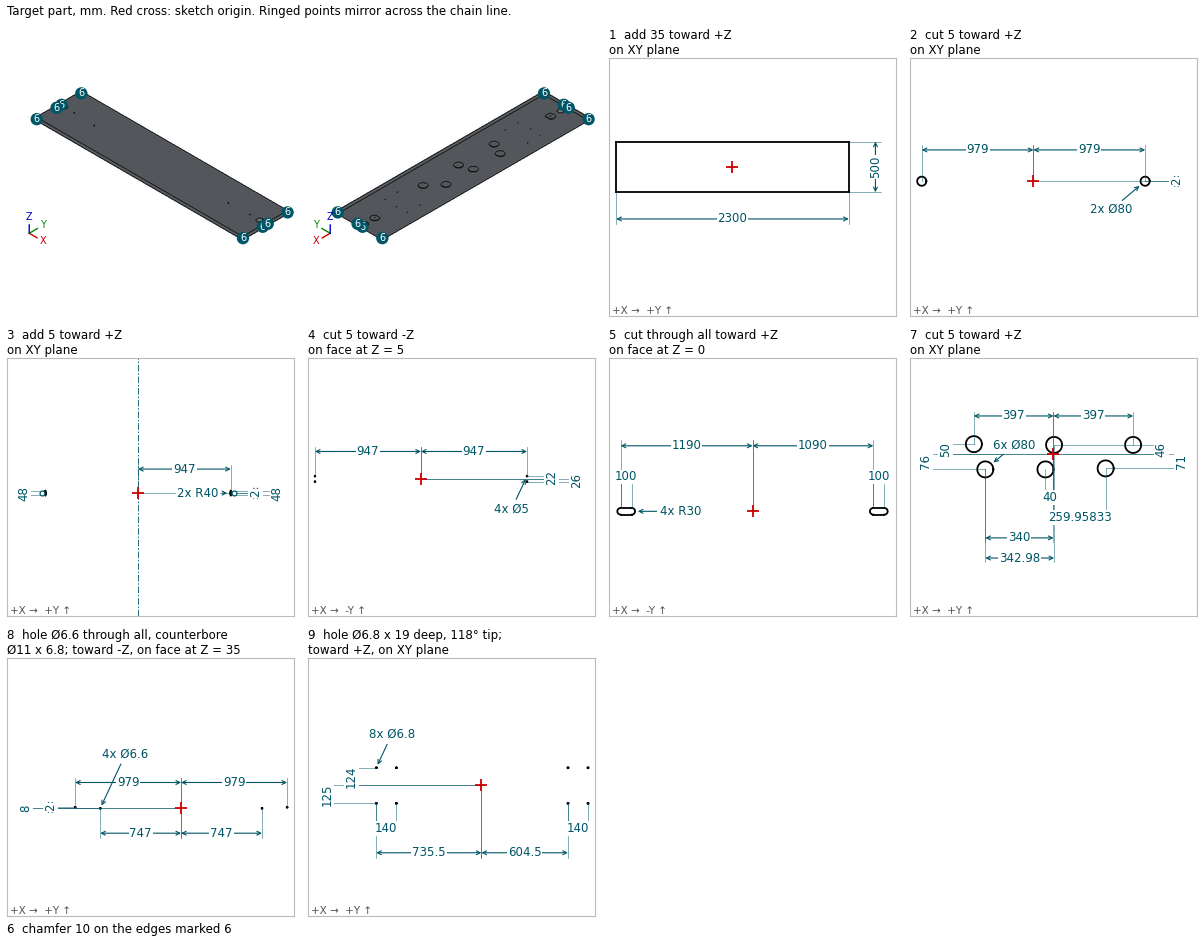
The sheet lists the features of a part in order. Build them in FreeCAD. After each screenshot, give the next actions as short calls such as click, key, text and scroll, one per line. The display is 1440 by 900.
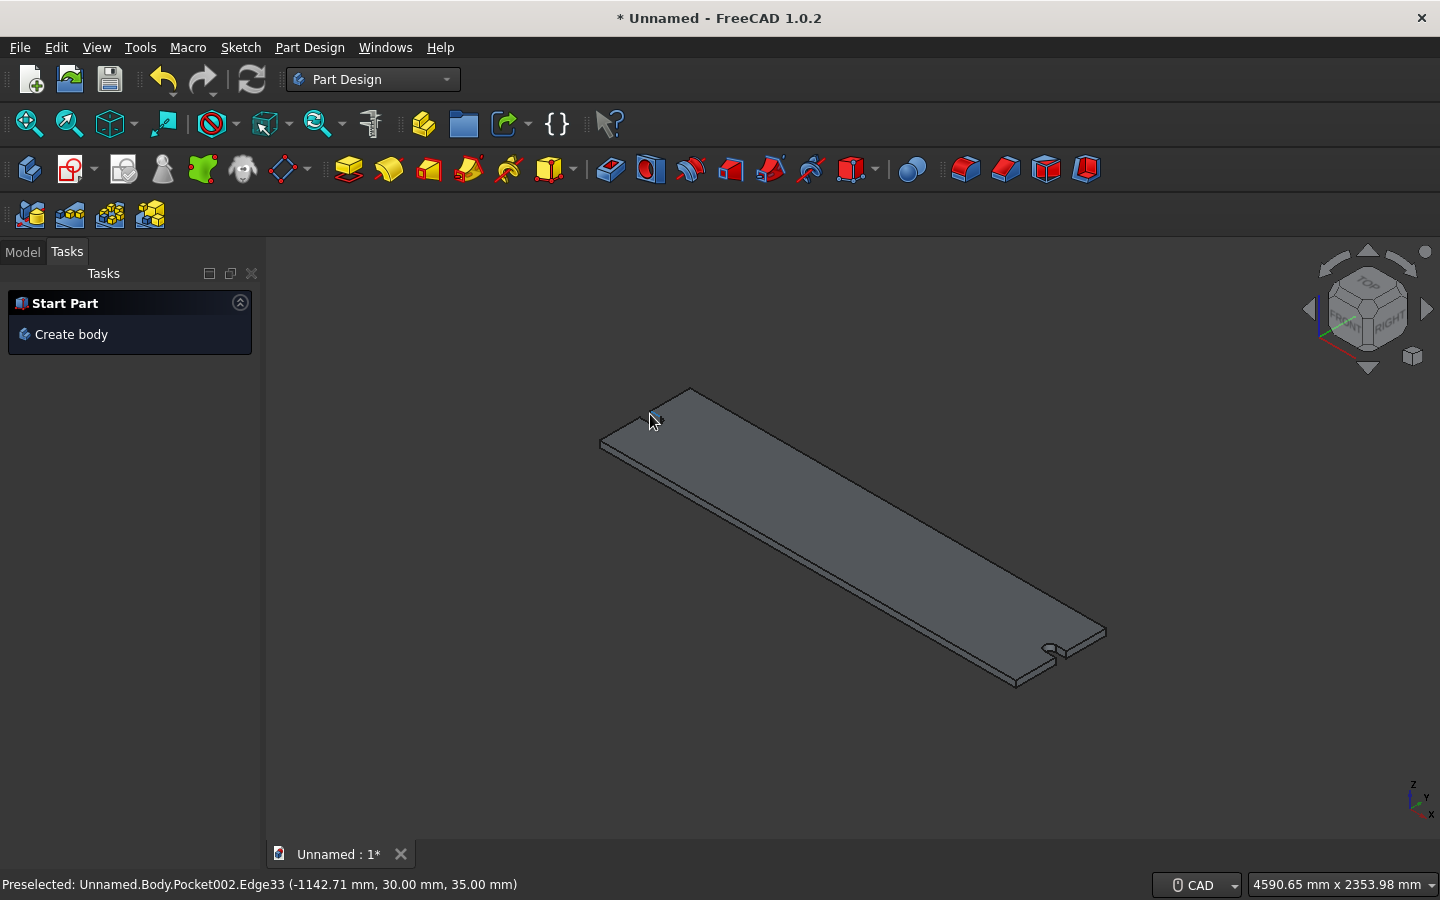
key(2)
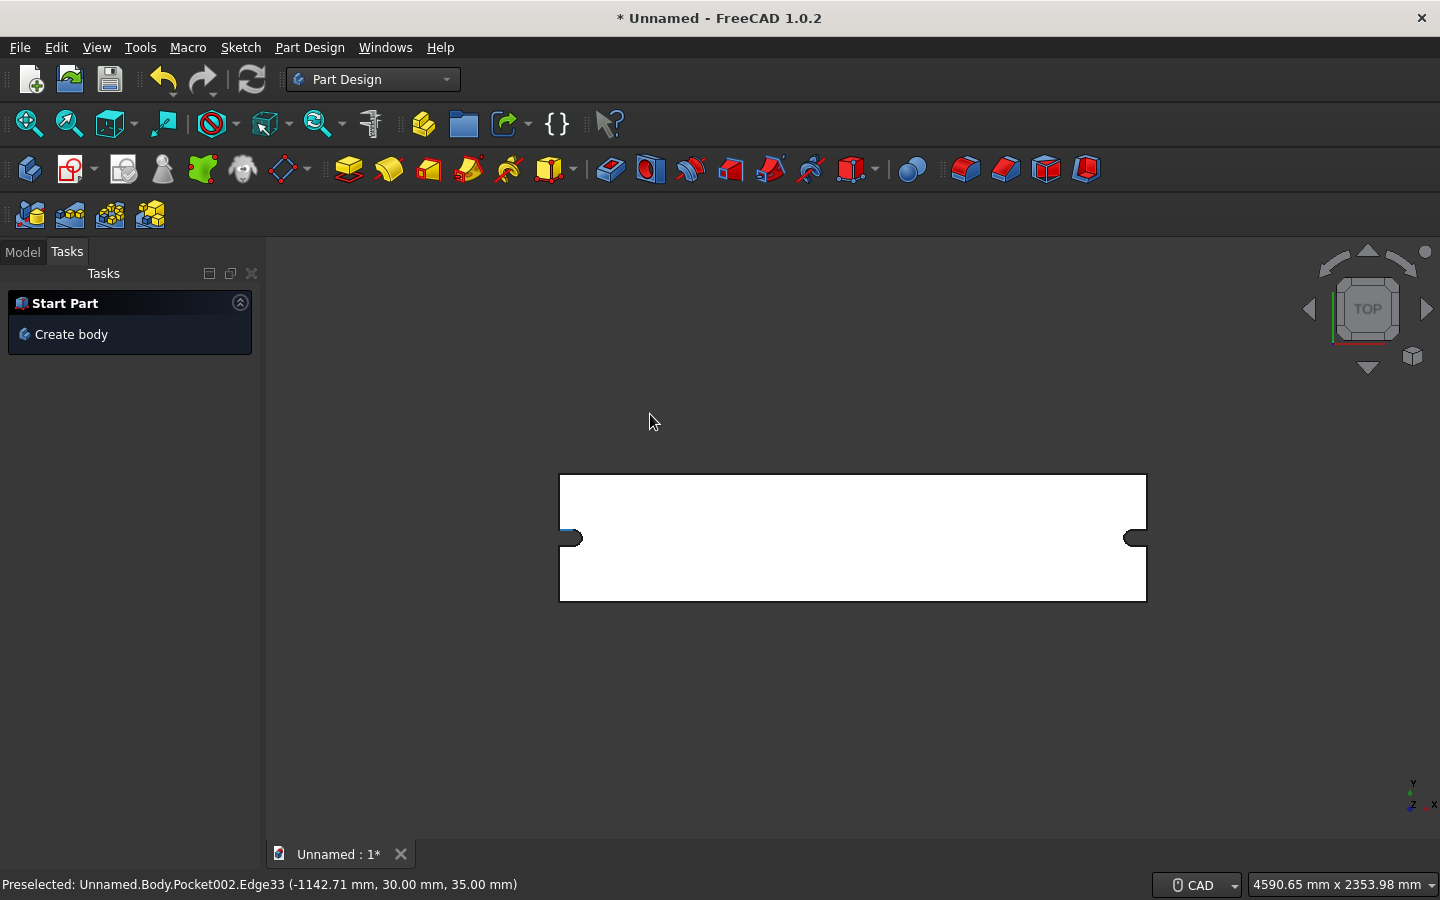
scroll(559, 529, up, 8)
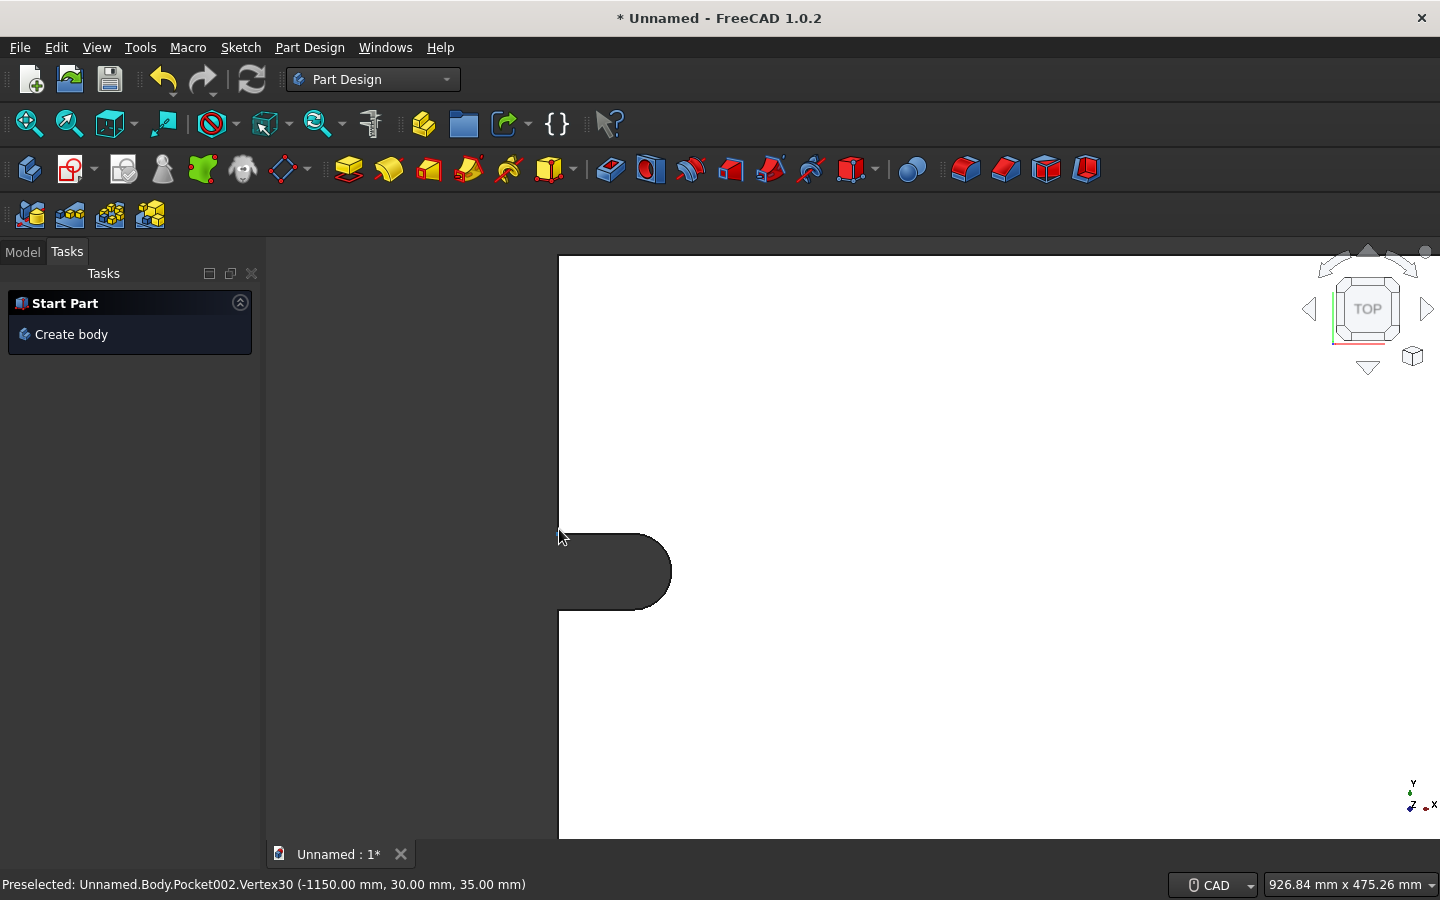
click(30, 124)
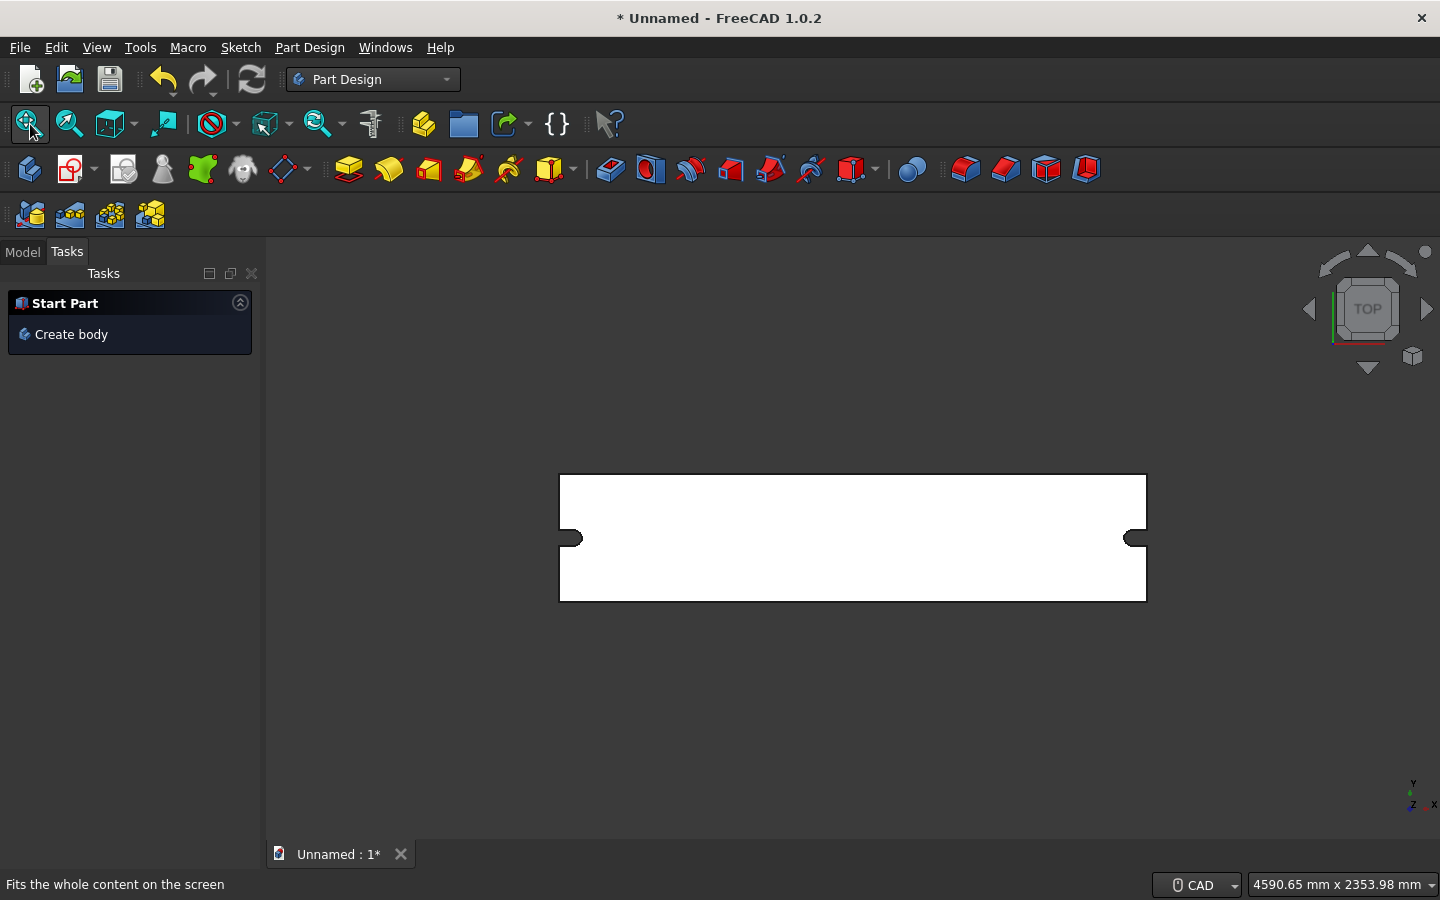
key(1)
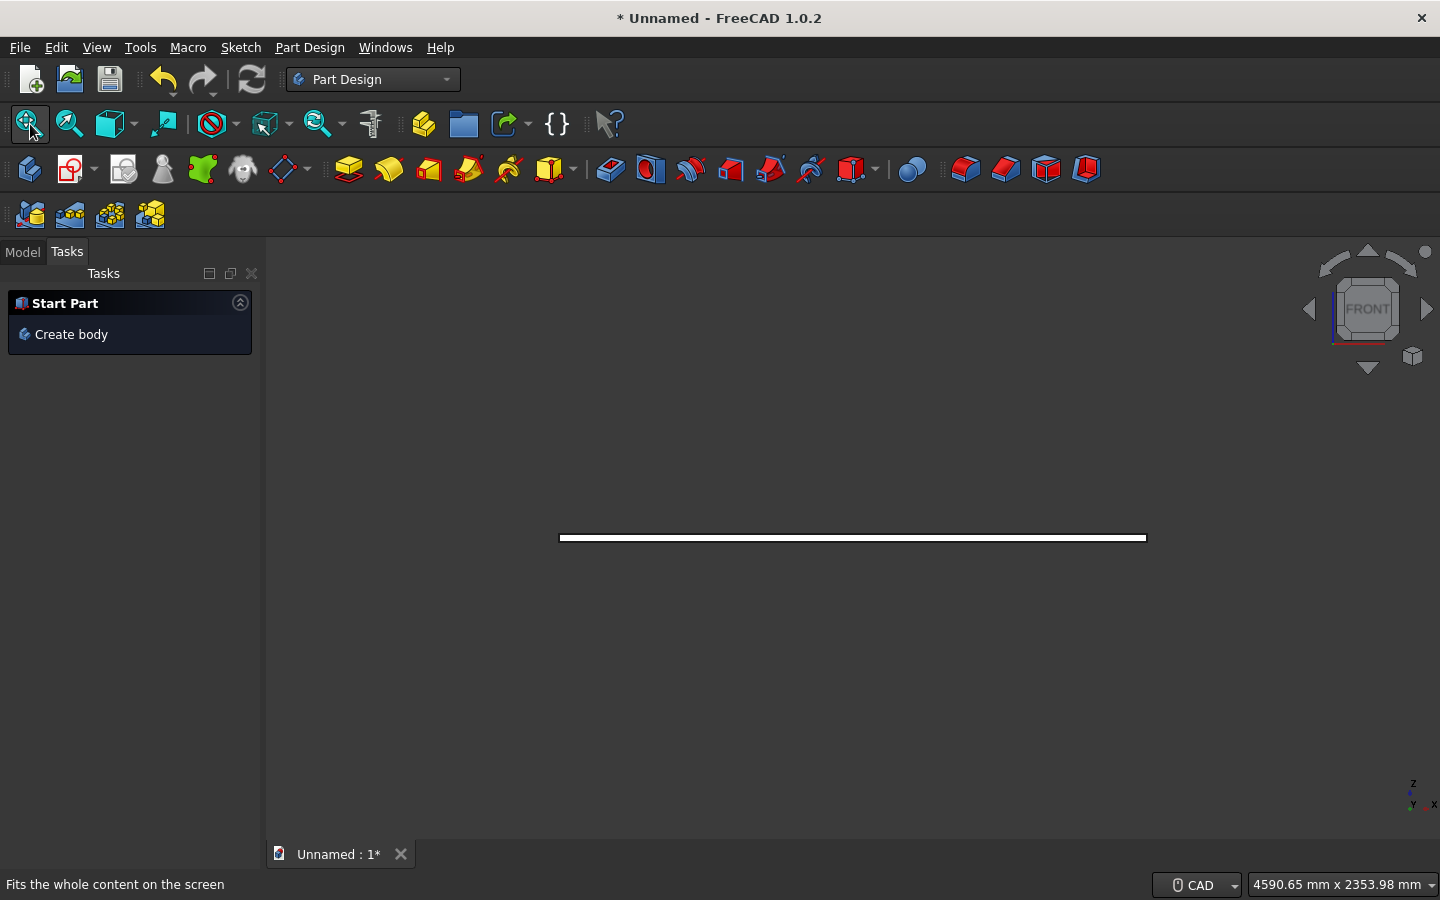
scroll(559, 537, up, 8)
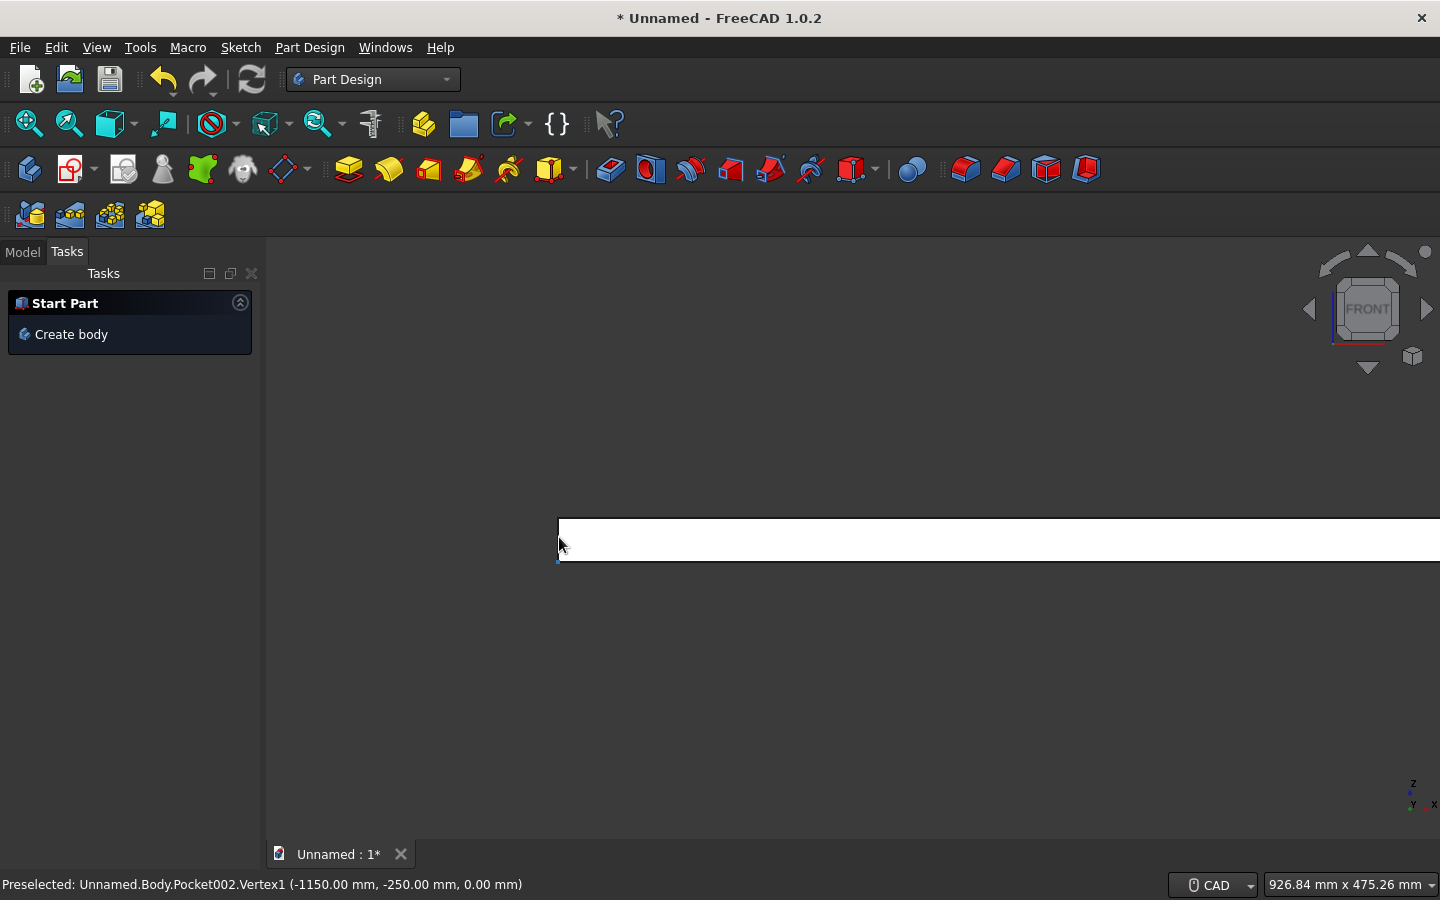
click(558, 539)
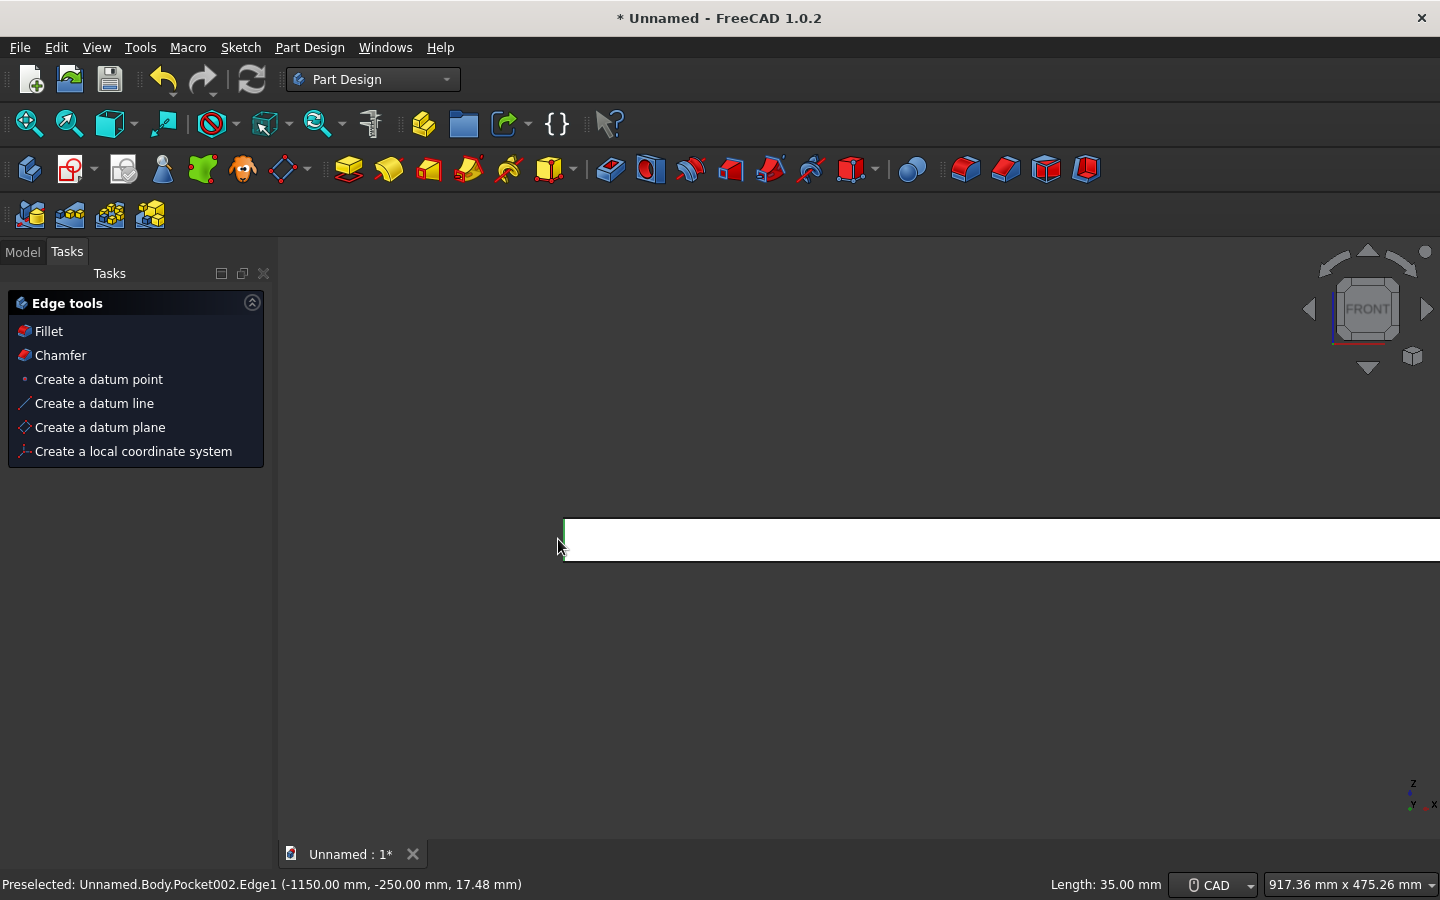
click(30, 124)